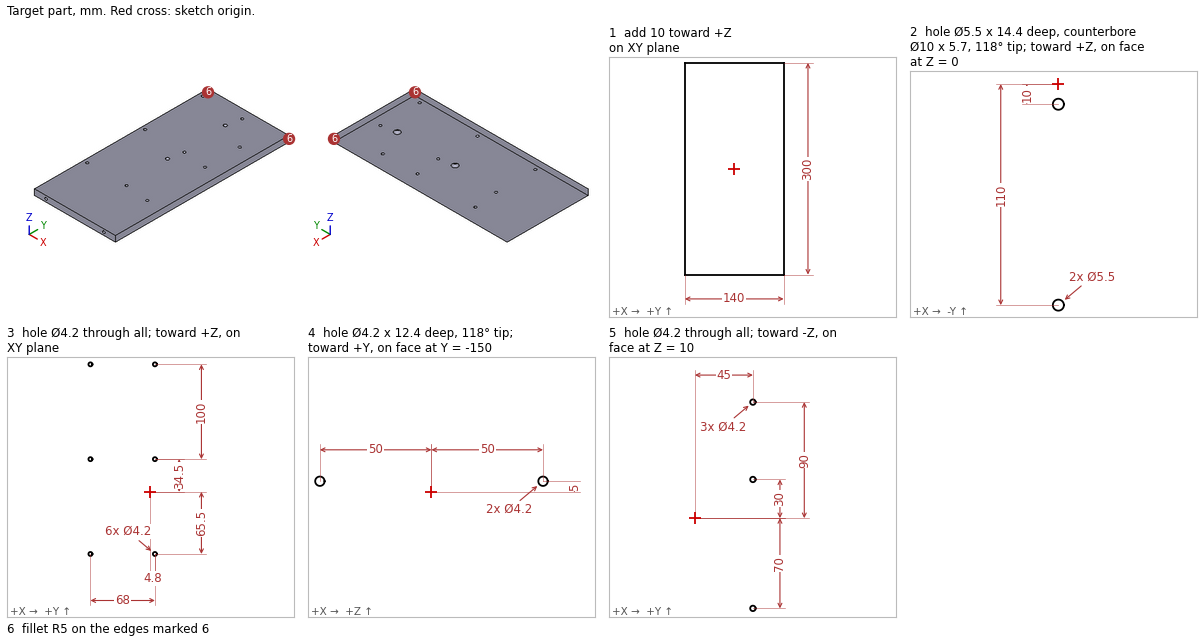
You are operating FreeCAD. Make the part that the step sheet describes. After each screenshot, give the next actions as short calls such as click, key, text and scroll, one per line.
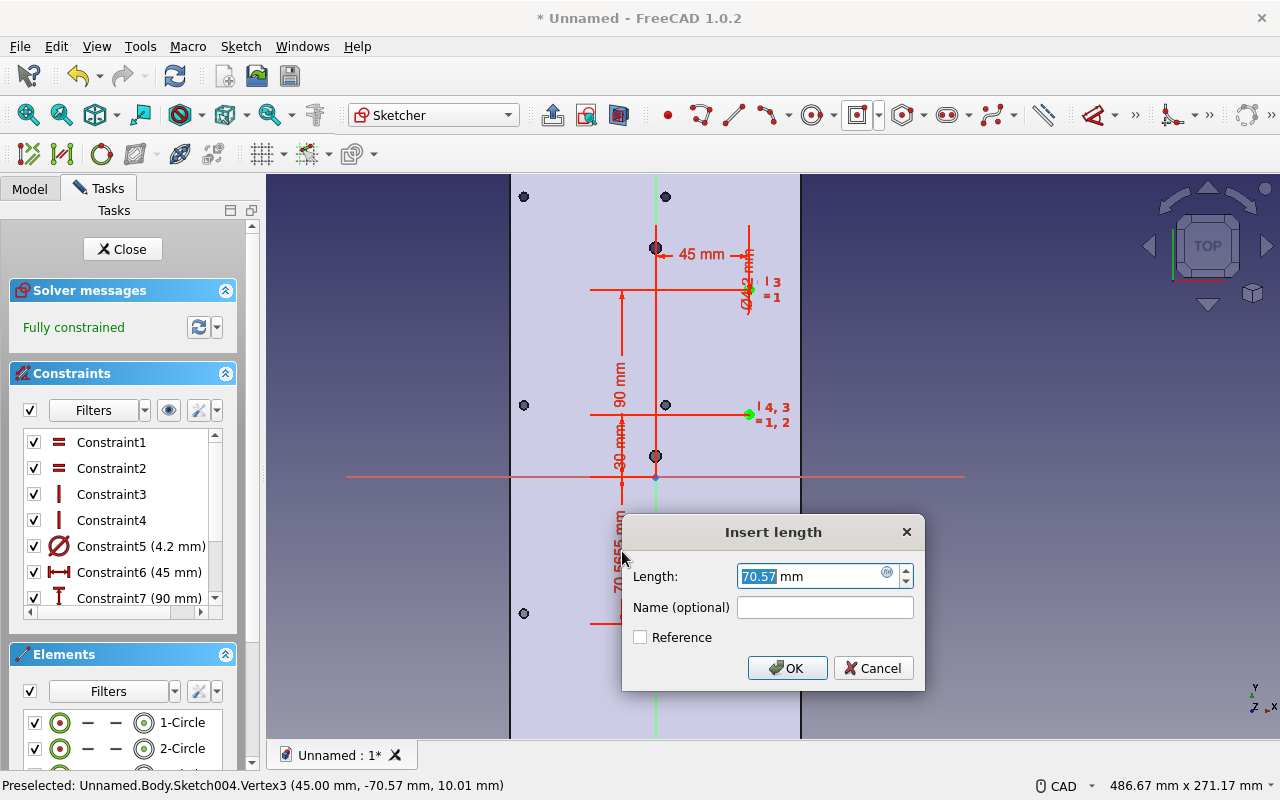
text(70)
key(Return)
key(Escape)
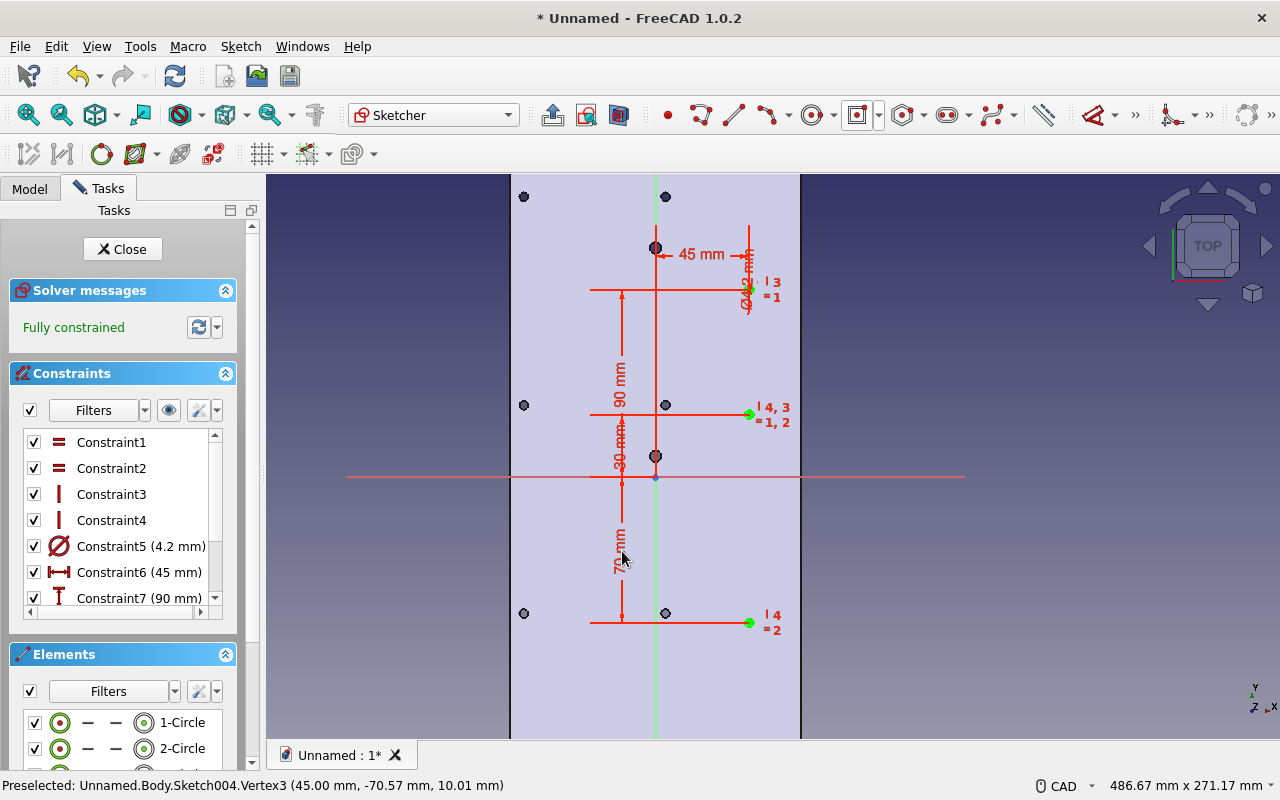
click(123, 249)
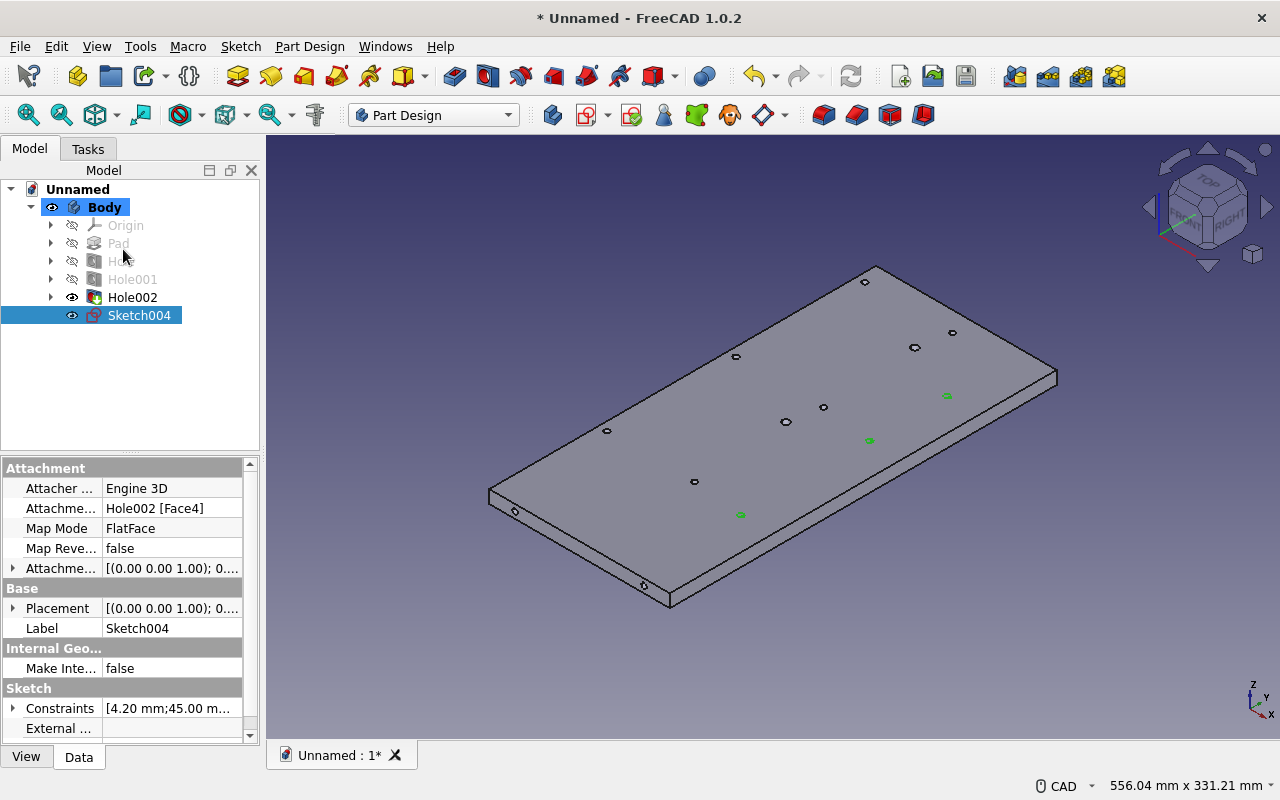
click(488, 76)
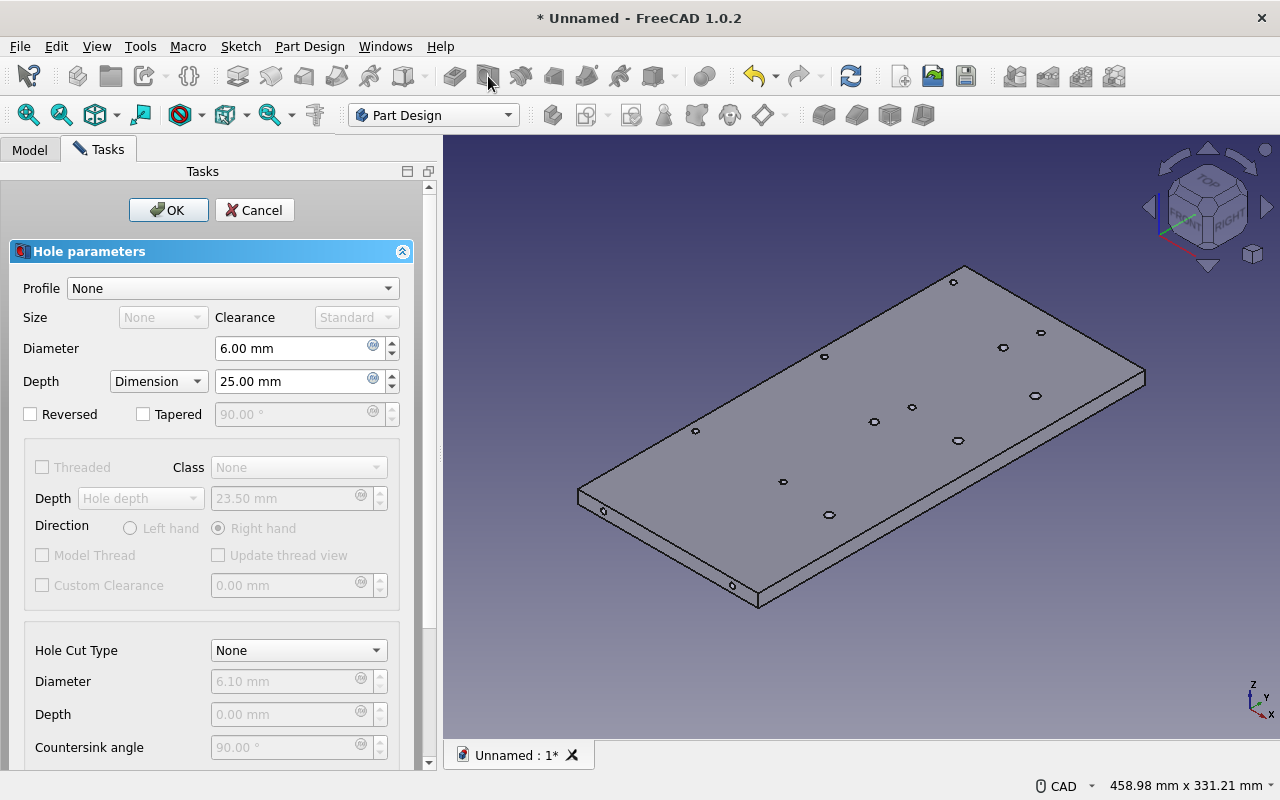
triple_click(300, 348)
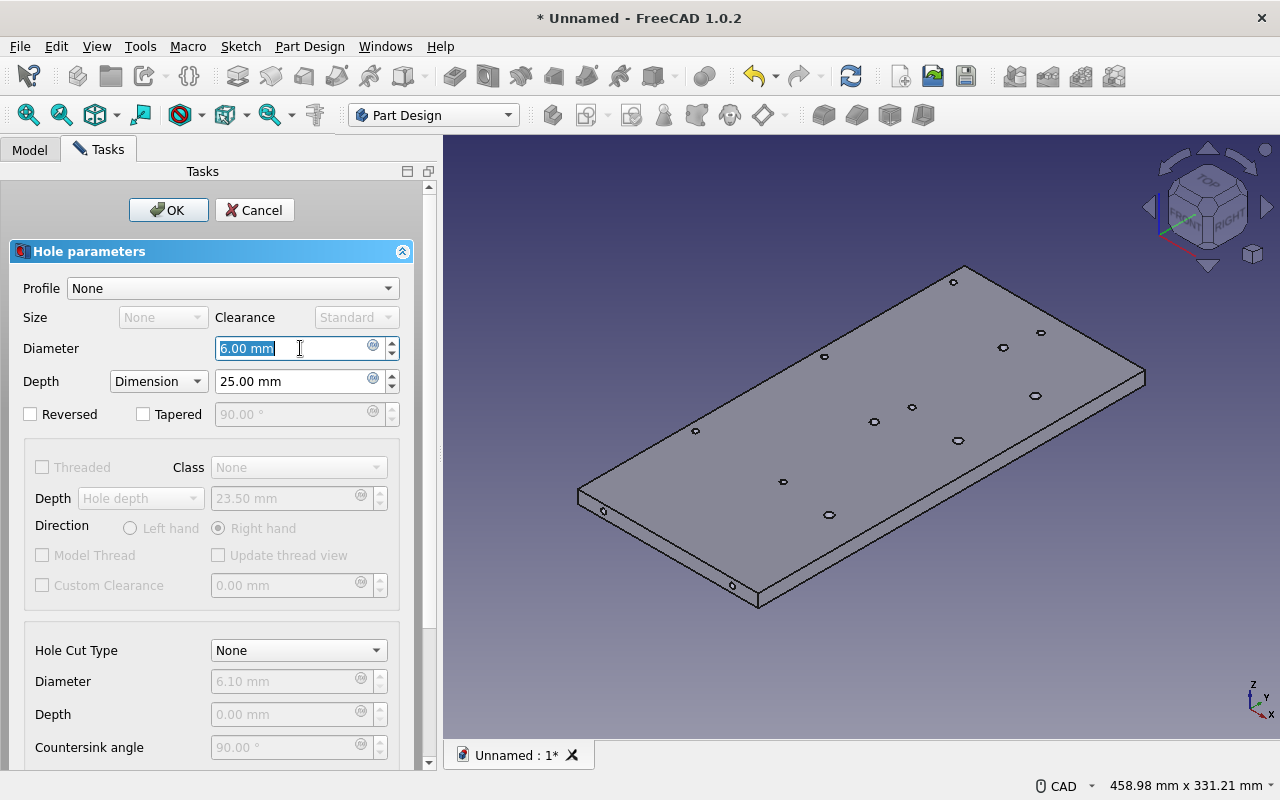
text(4.2)
key(Tab)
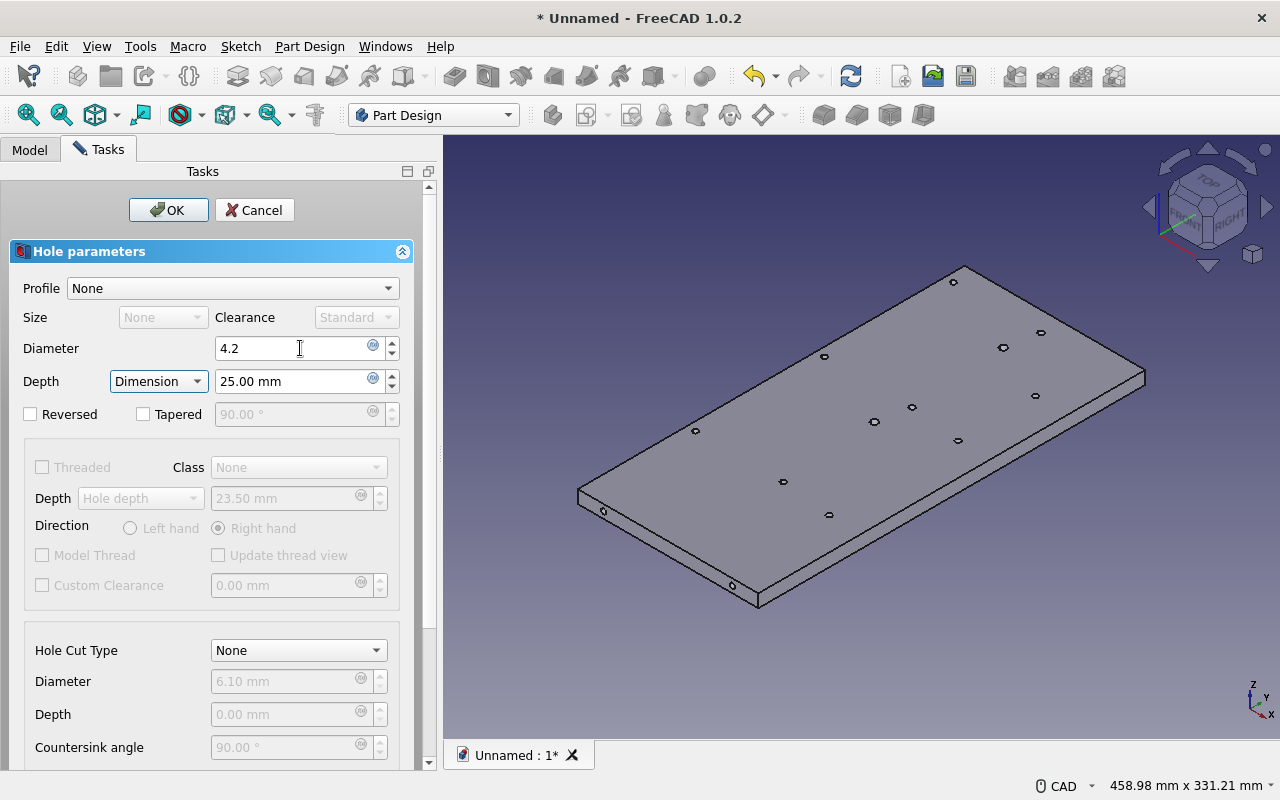
click(160, 382)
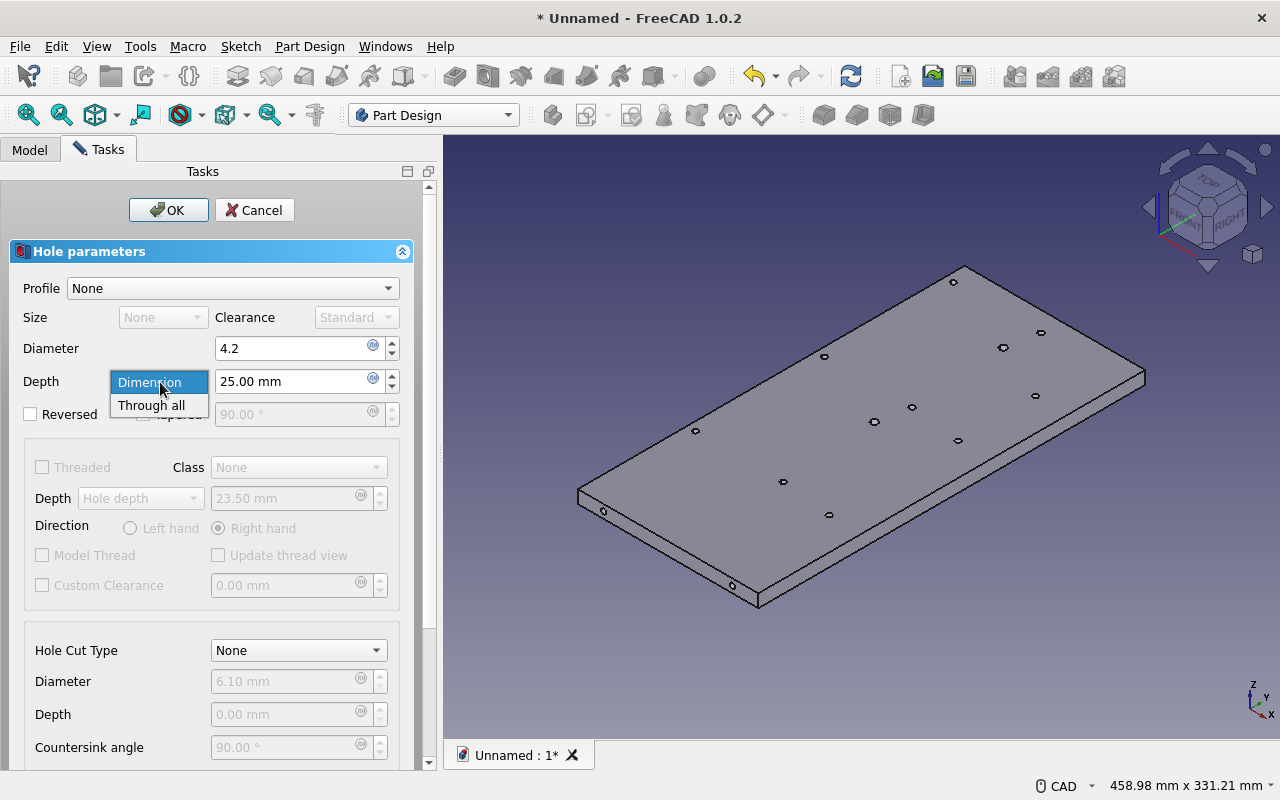
click(158, 406)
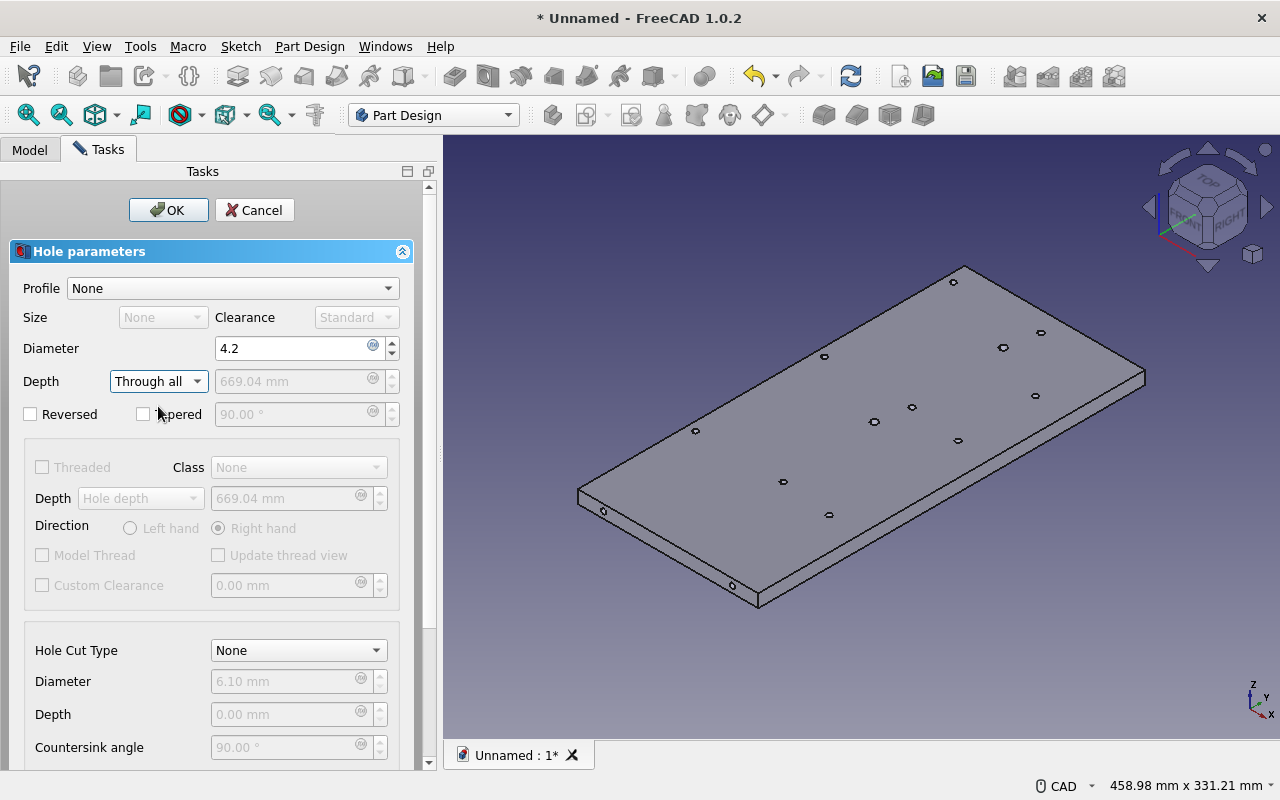
click(169, 210)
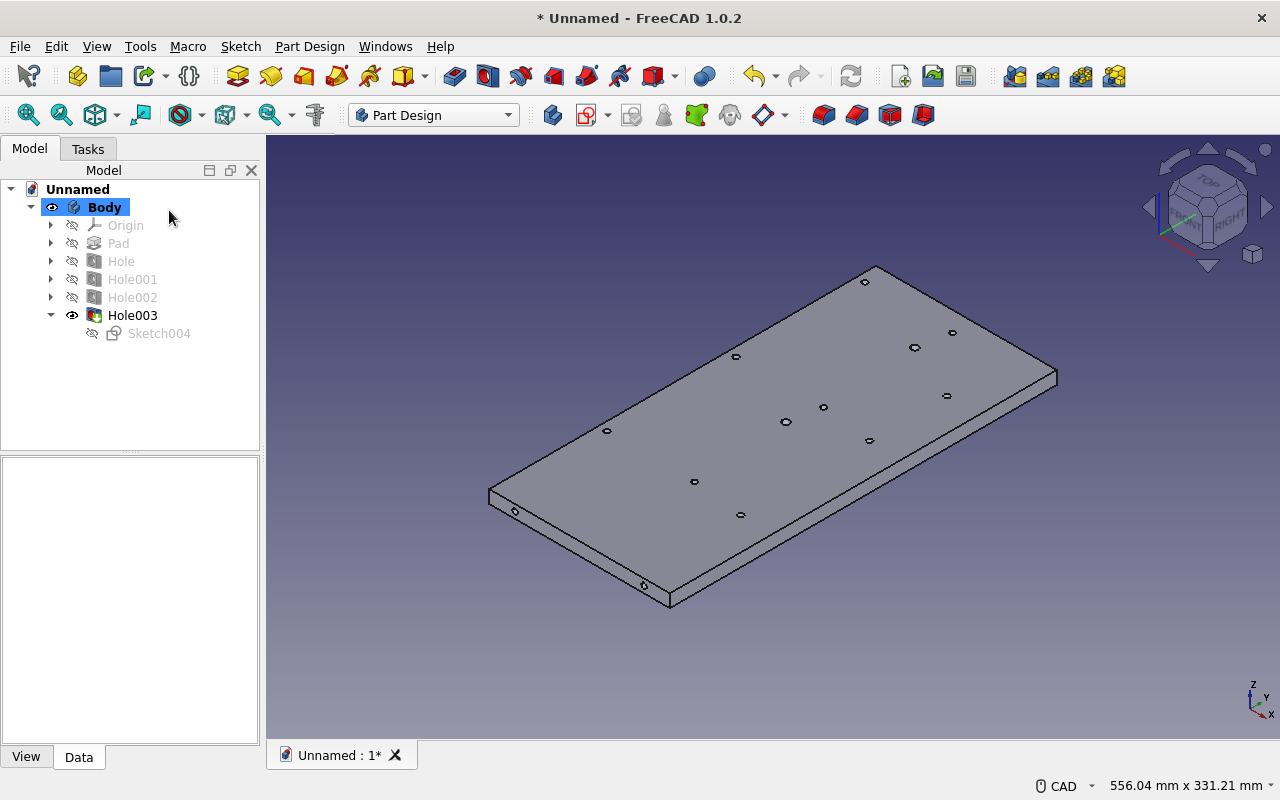
scroll(876, 272, up, 4)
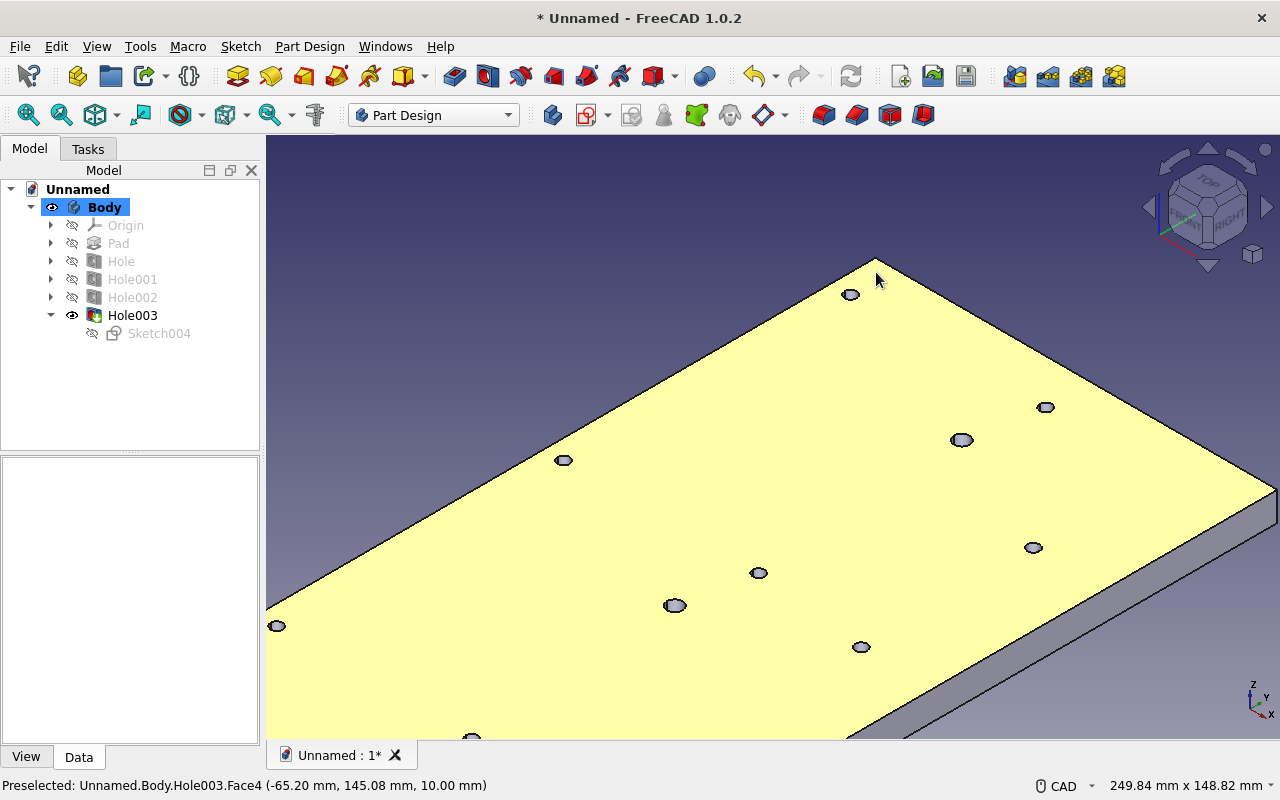
click(29, 116)